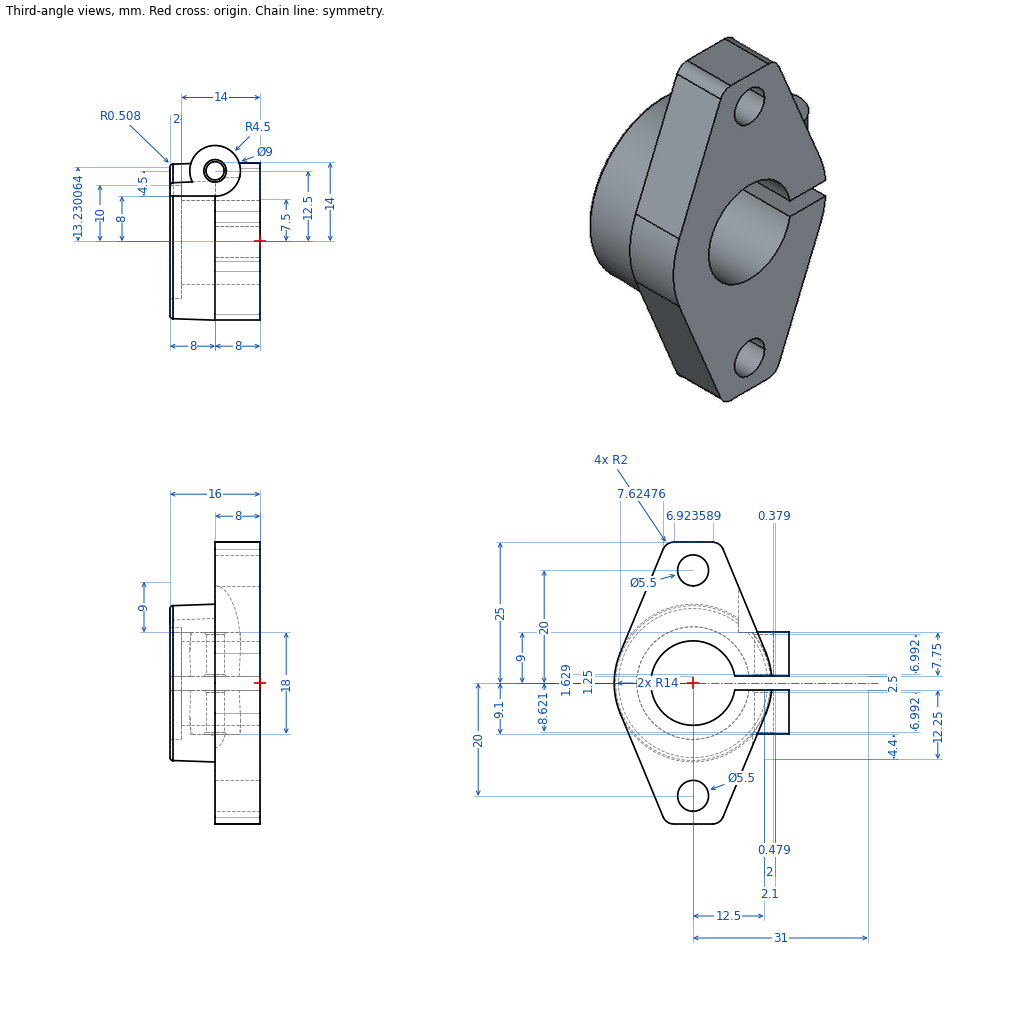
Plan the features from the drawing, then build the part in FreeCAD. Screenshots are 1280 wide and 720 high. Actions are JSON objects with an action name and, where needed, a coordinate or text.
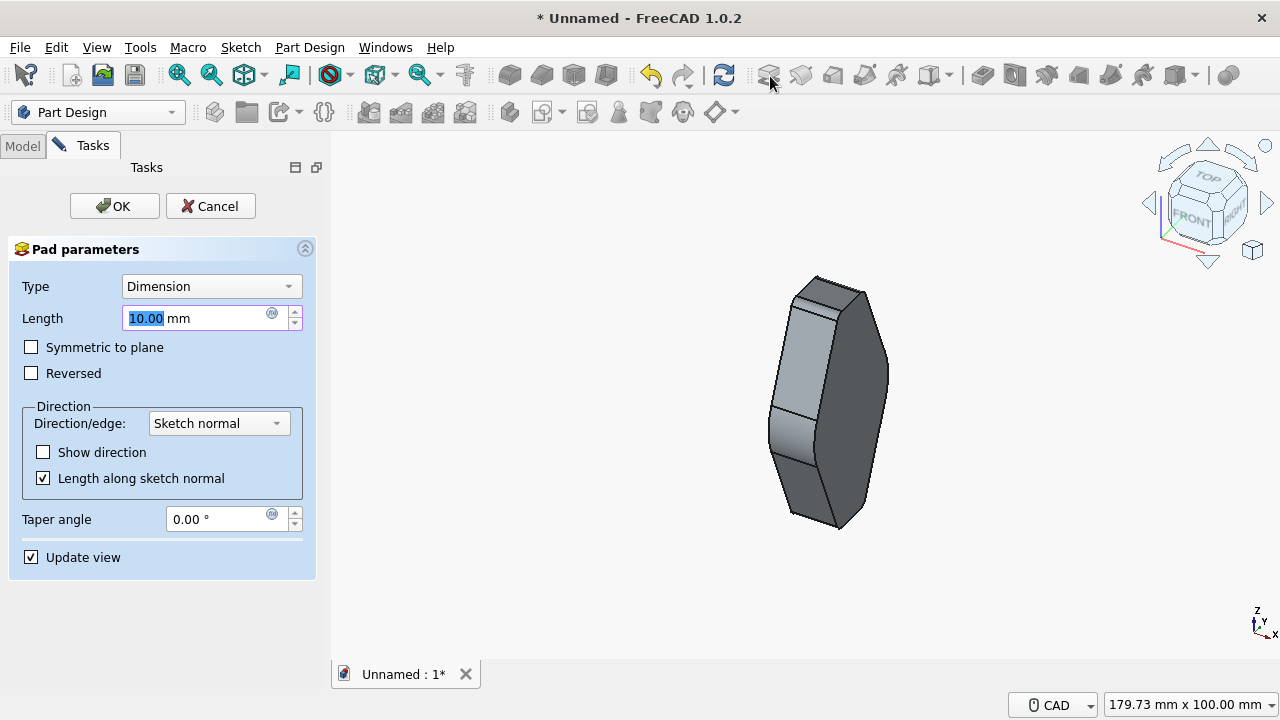
{"action": "type", "text": "8"}
{"action": "key", "text": "Tab"}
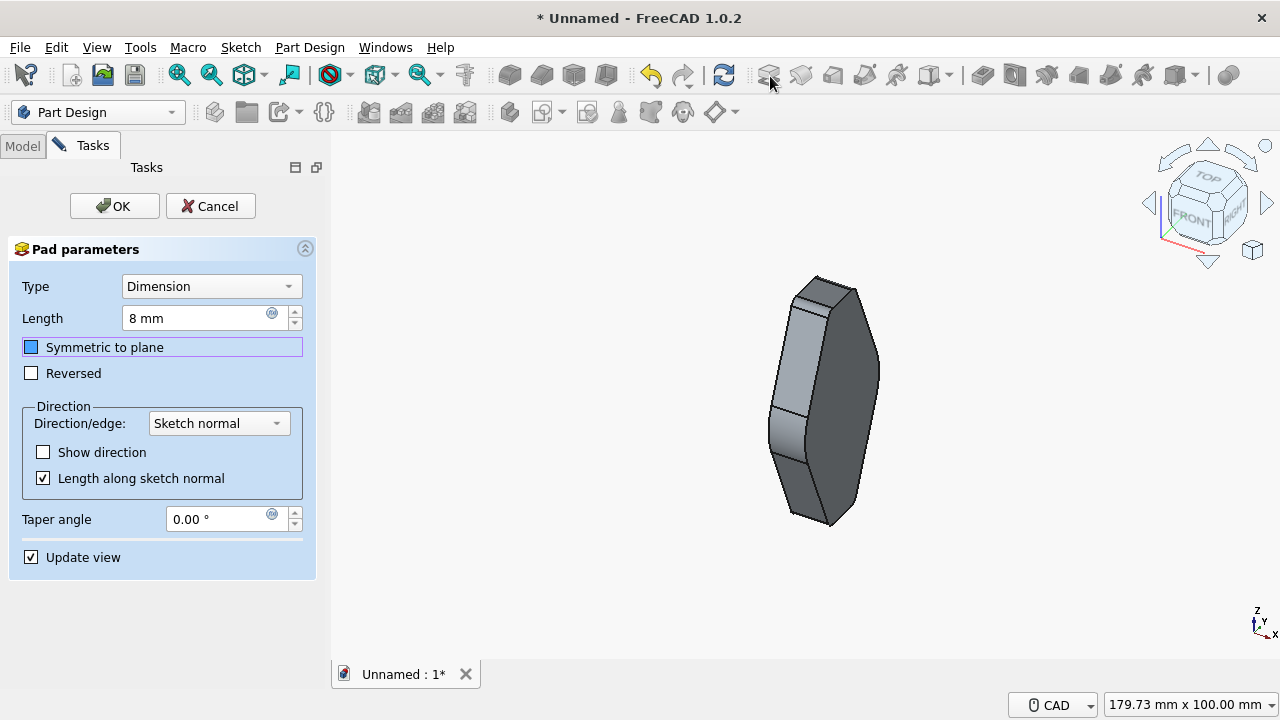
{"action": "left_click", "coordinate": [30, 373]}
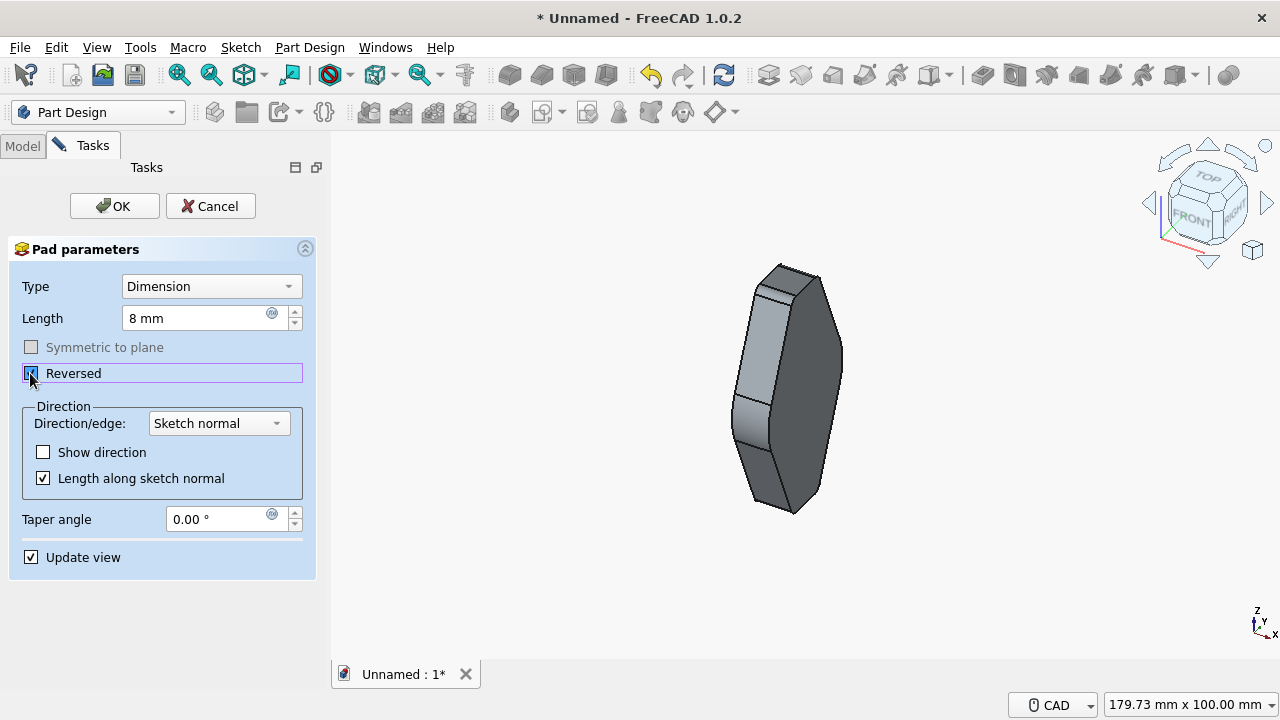
{"action": "left_click", "coordinate": [115, 206]}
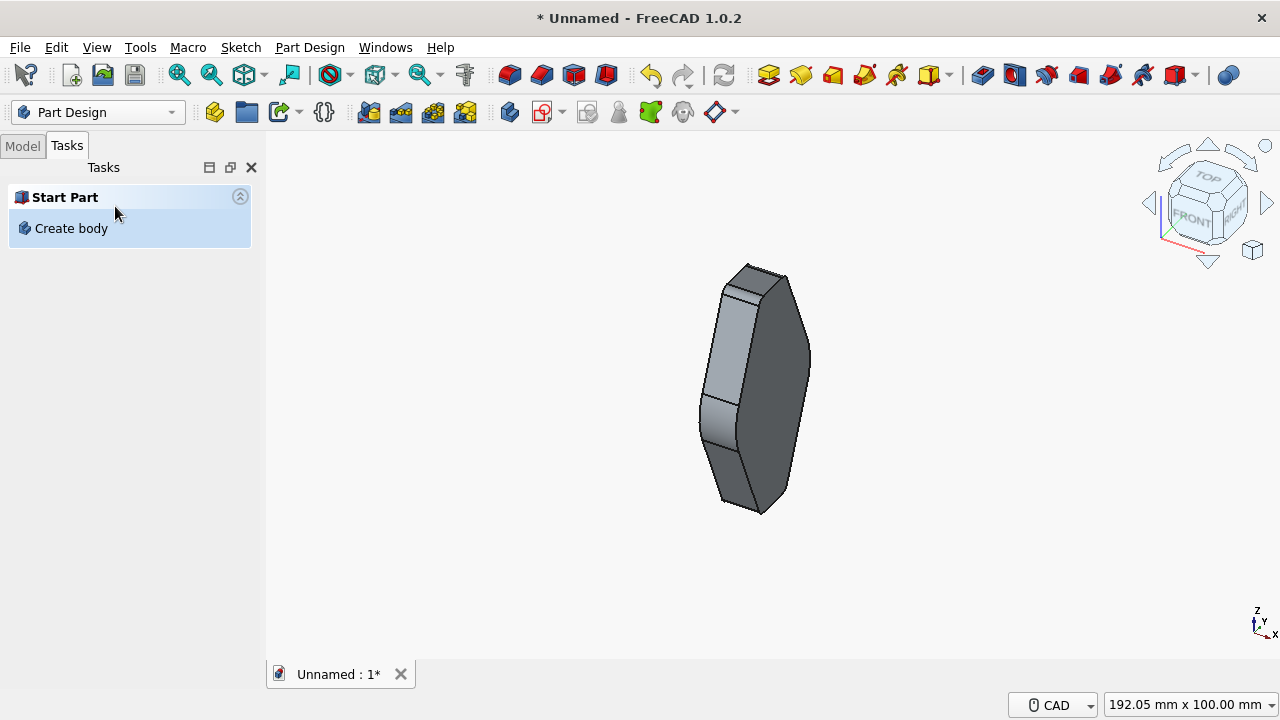
{"action": "left_click", "coordinate": [542, 112]}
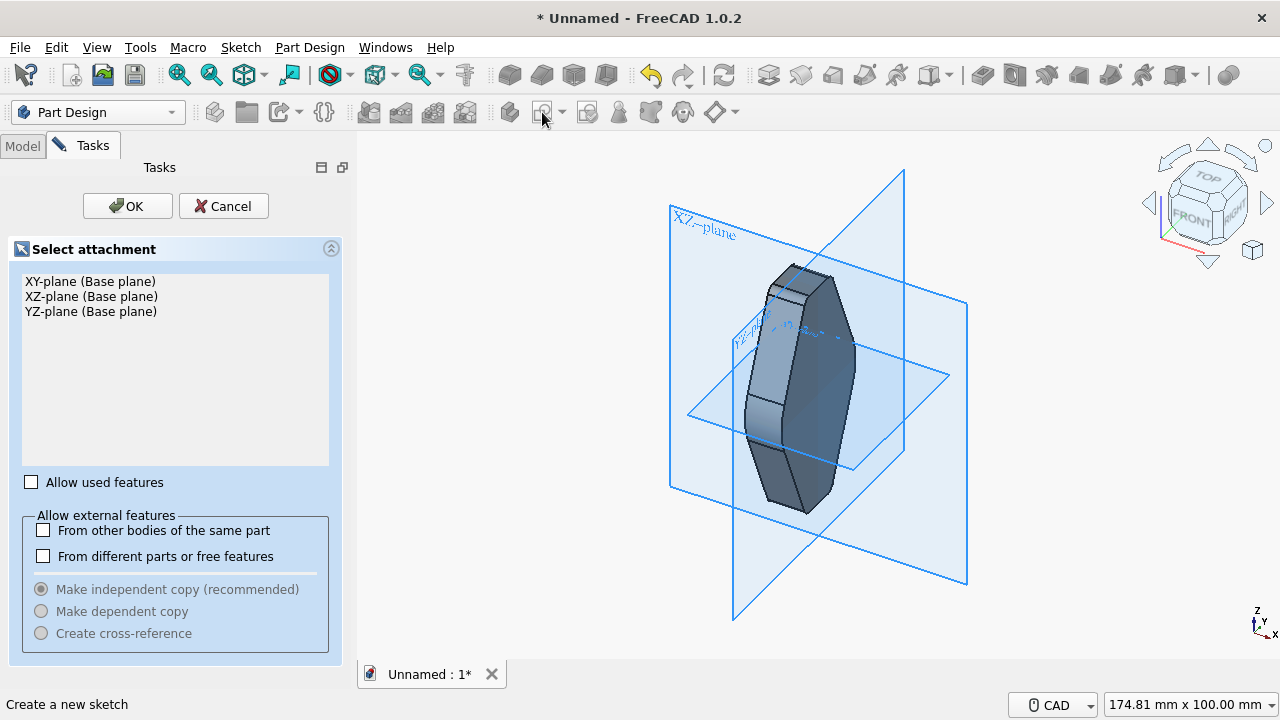
{"action": "left_click", "coordinate": [82, 282]}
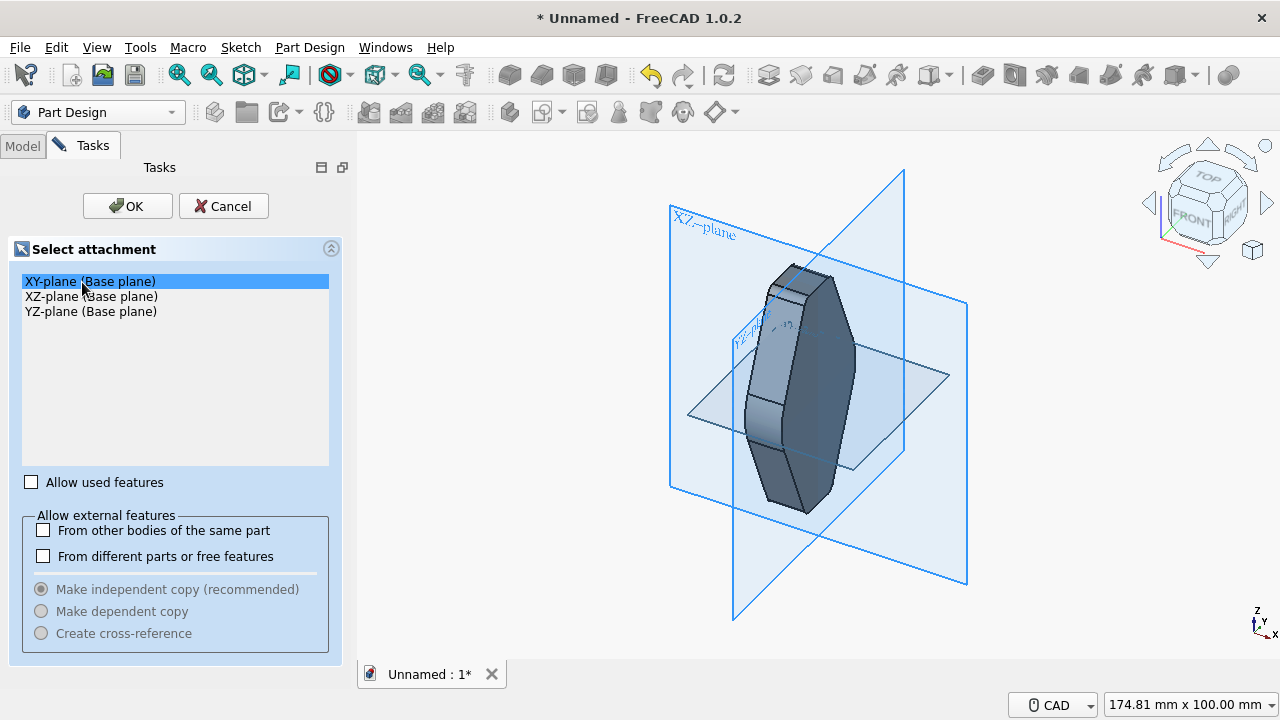
{"action": "left_click", "coordinate": [128, 206]}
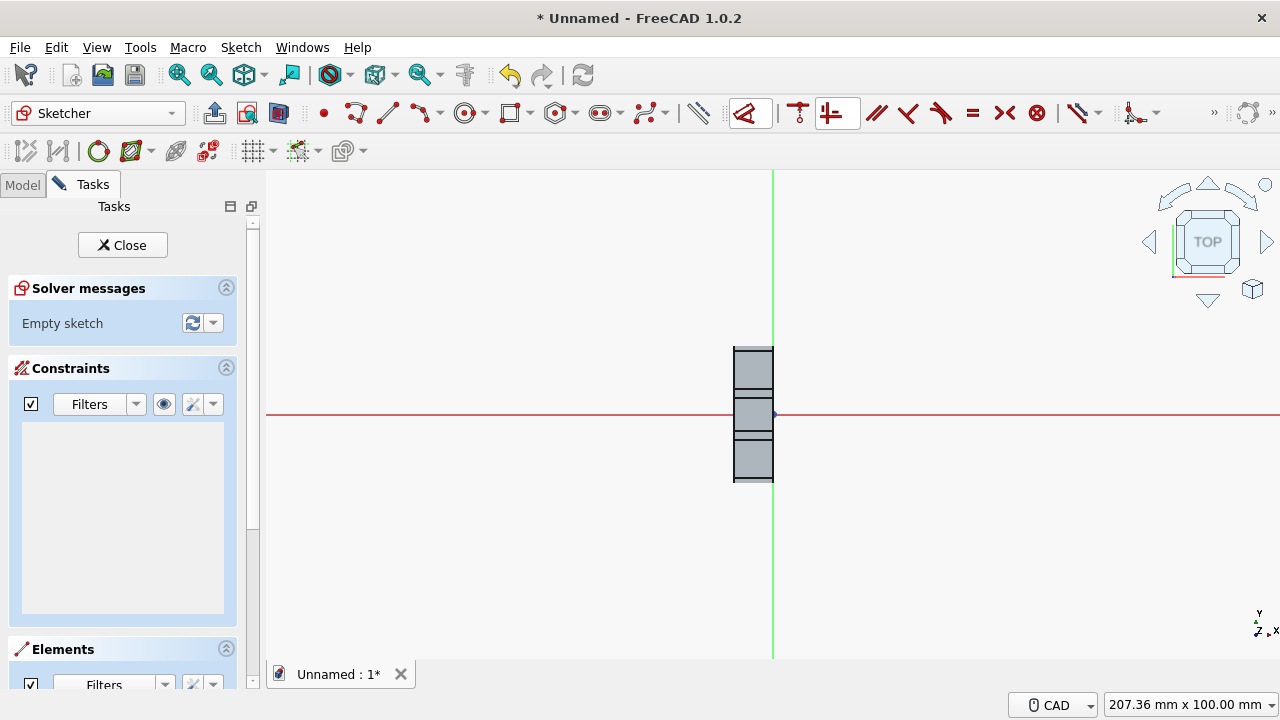
{"action": "left_click", "coordinate": [280, 114]}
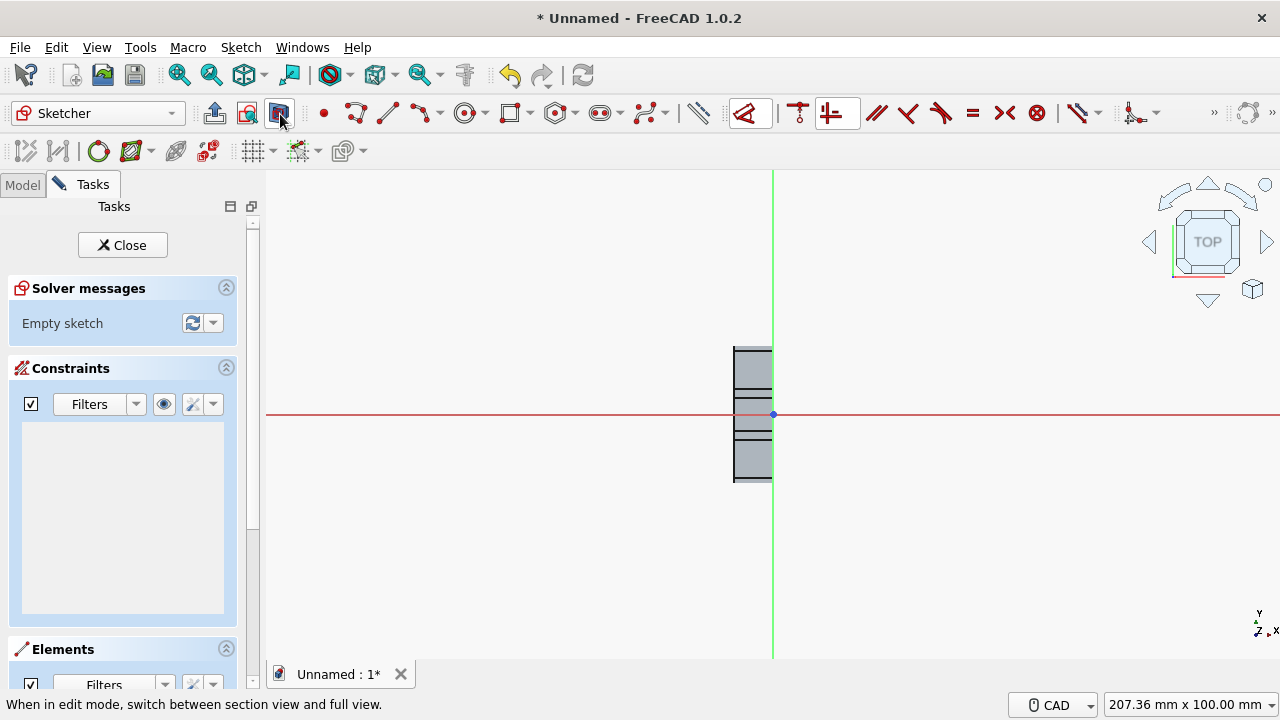
{"action": "scroll", "coordinate": [743, 369], "scroll_direction": "up", "scroll_amount": 7}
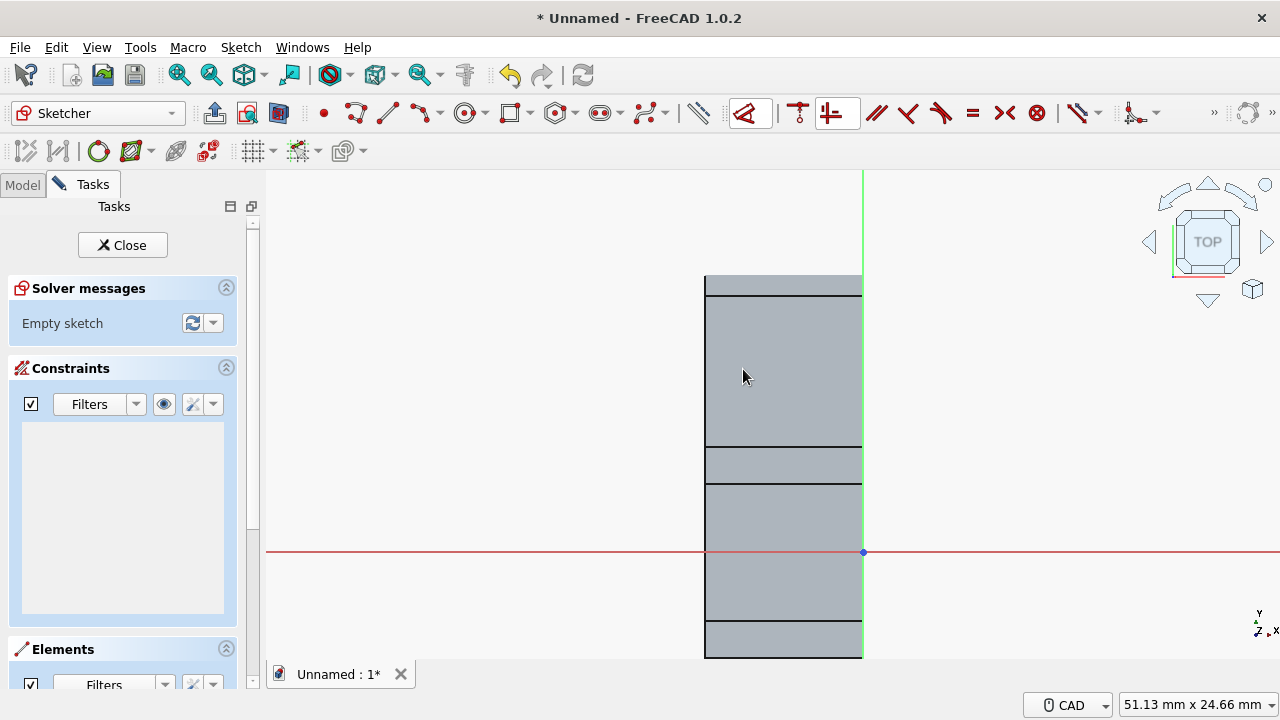
{"action": "left_click", "coordinate": [356, 114]}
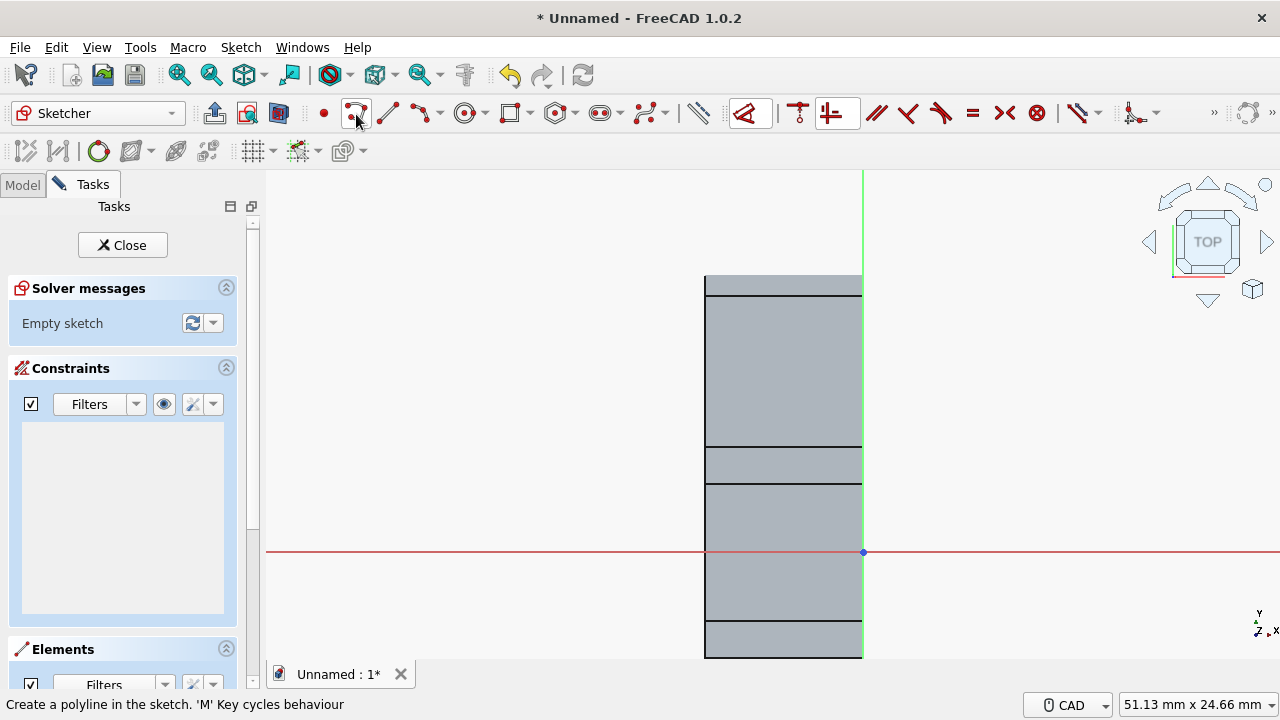
{"action": "left_click", "coordinate": [546, 290]}
{"action": "left_click", "coordinate": [546, 552]}
{"action": "left_click", "coordinate": [705, 543]}
{"action": "left_click", "coordinate": [705, 275]}
{"action": "left_click", "coordinate": [556, 283]}
{"action": "right_click", "coordinate": [556, 283]}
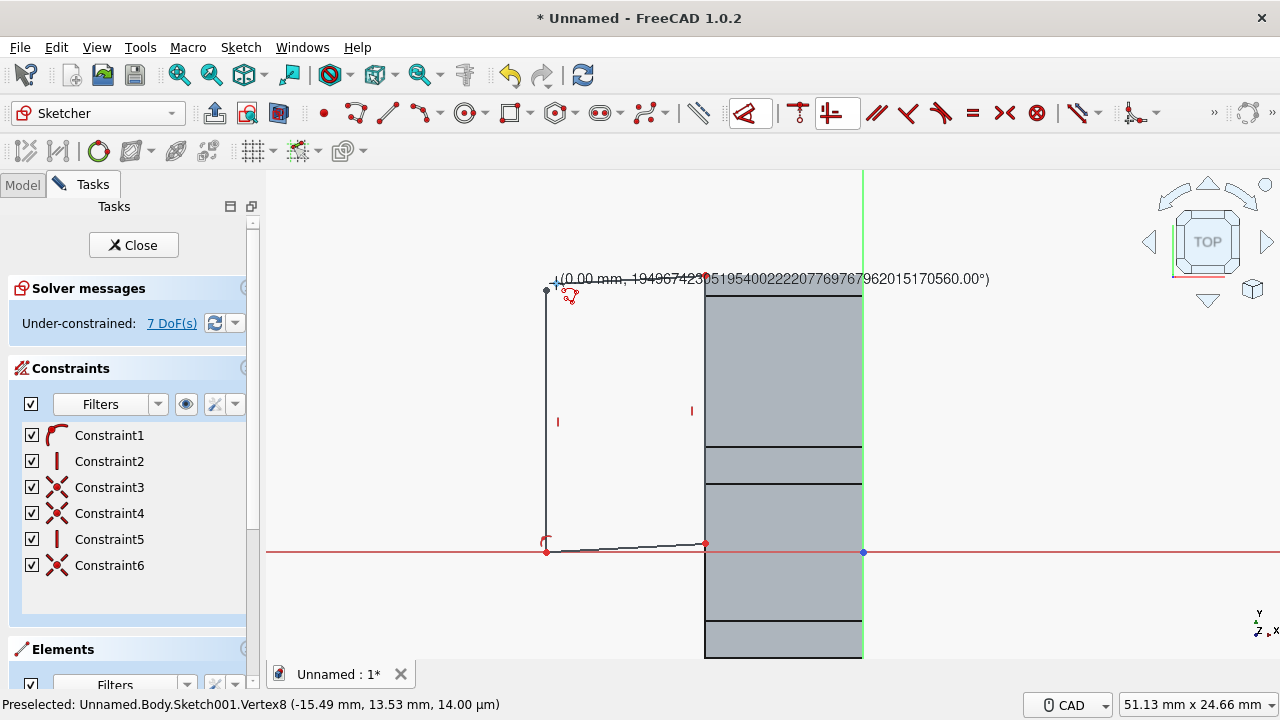
{"action": "left_click", "coordinate": [420, 114]}